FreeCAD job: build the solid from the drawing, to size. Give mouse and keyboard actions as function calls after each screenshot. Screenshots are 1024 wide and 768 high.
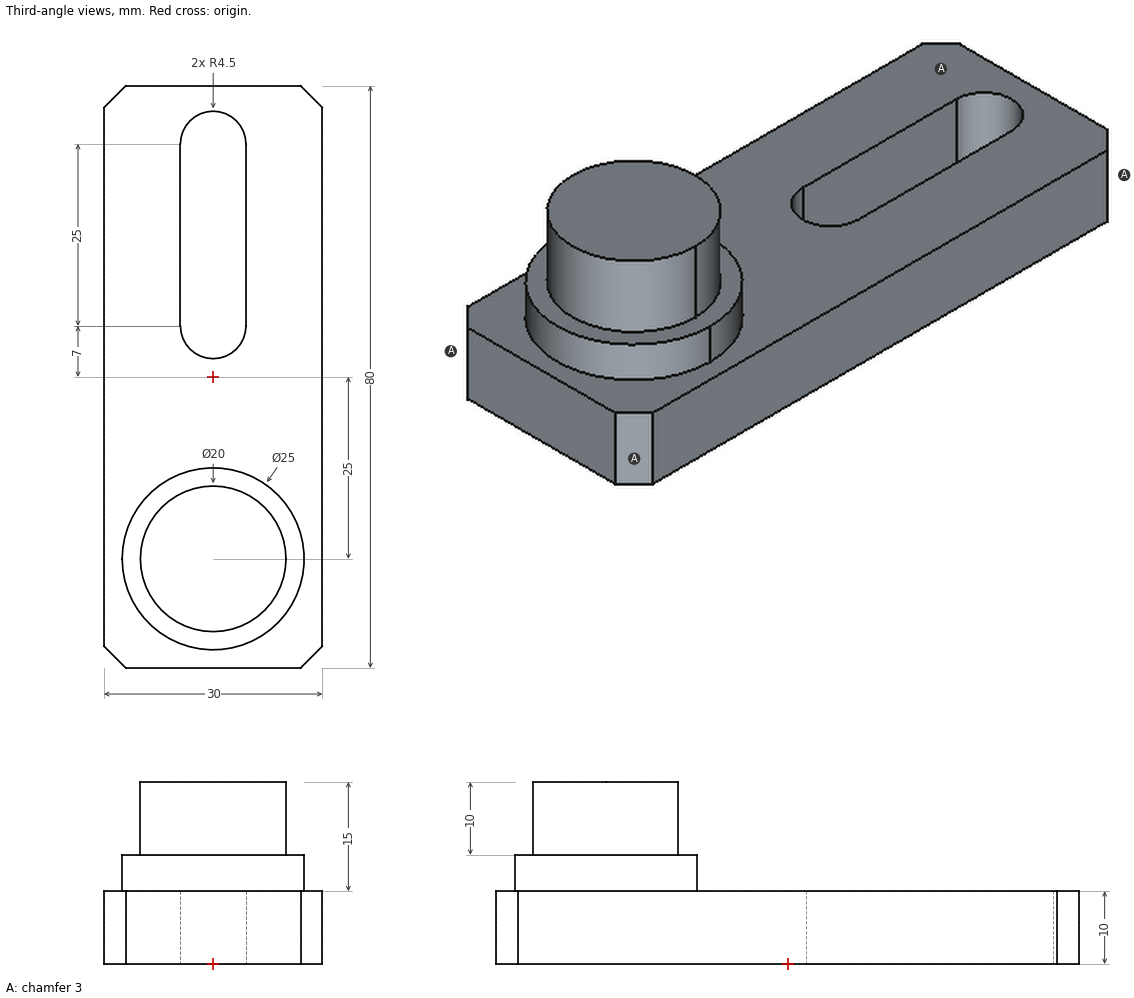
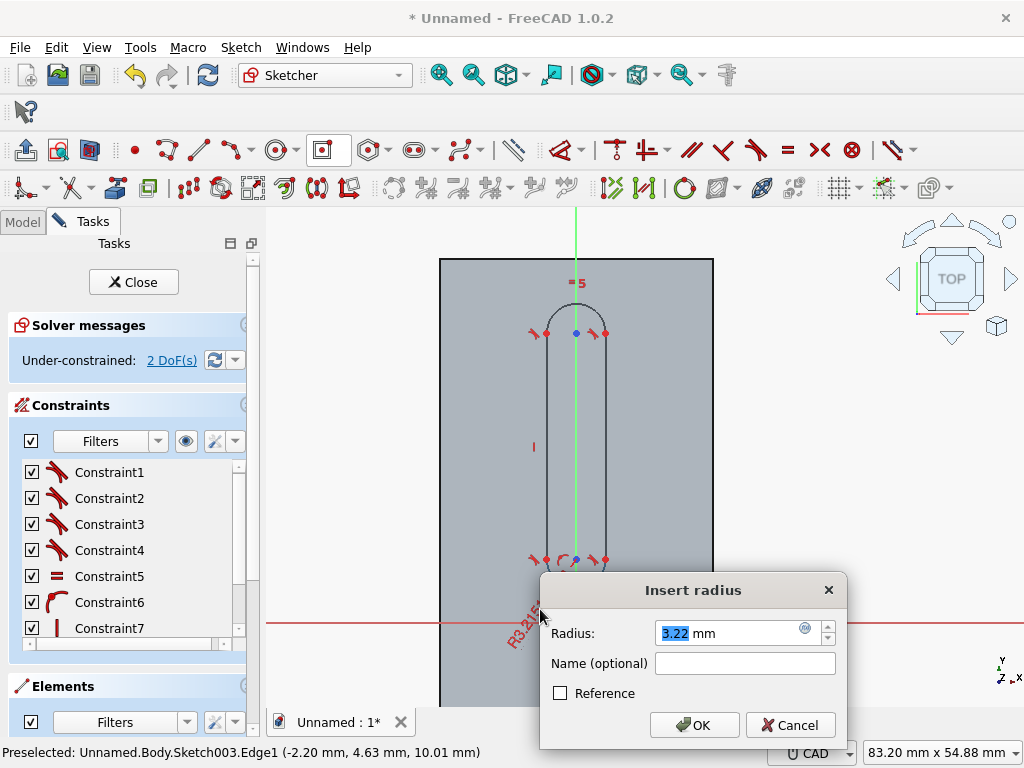
text(4.5)
key(Return)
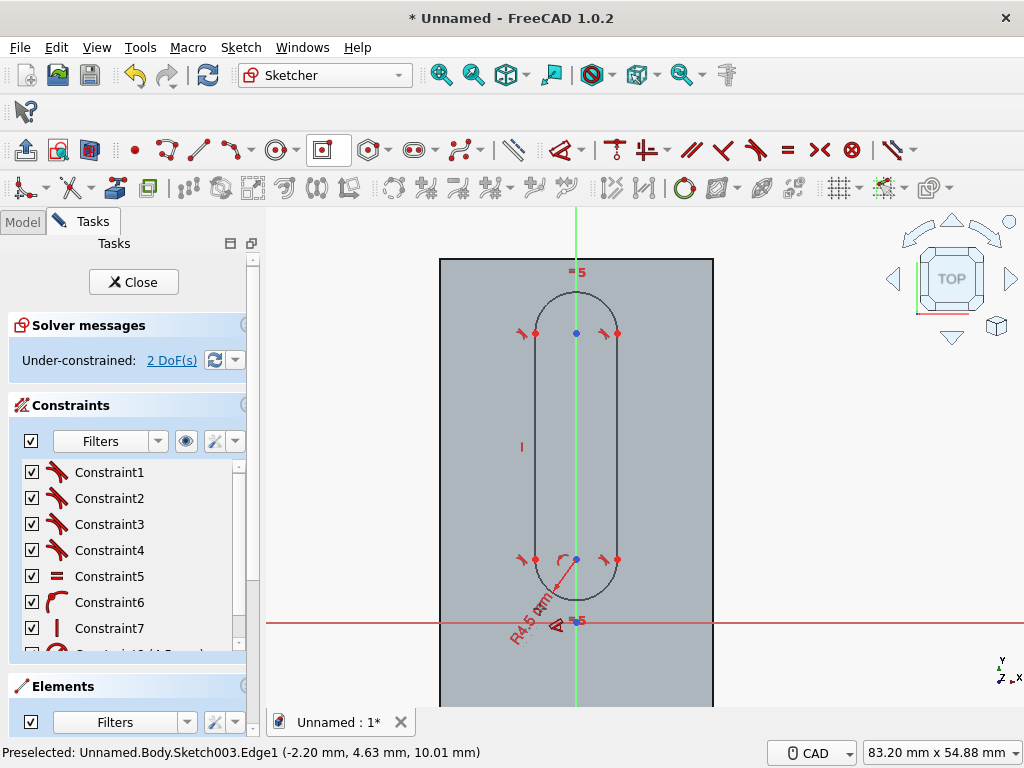
click(535, 492)
click(501, 446)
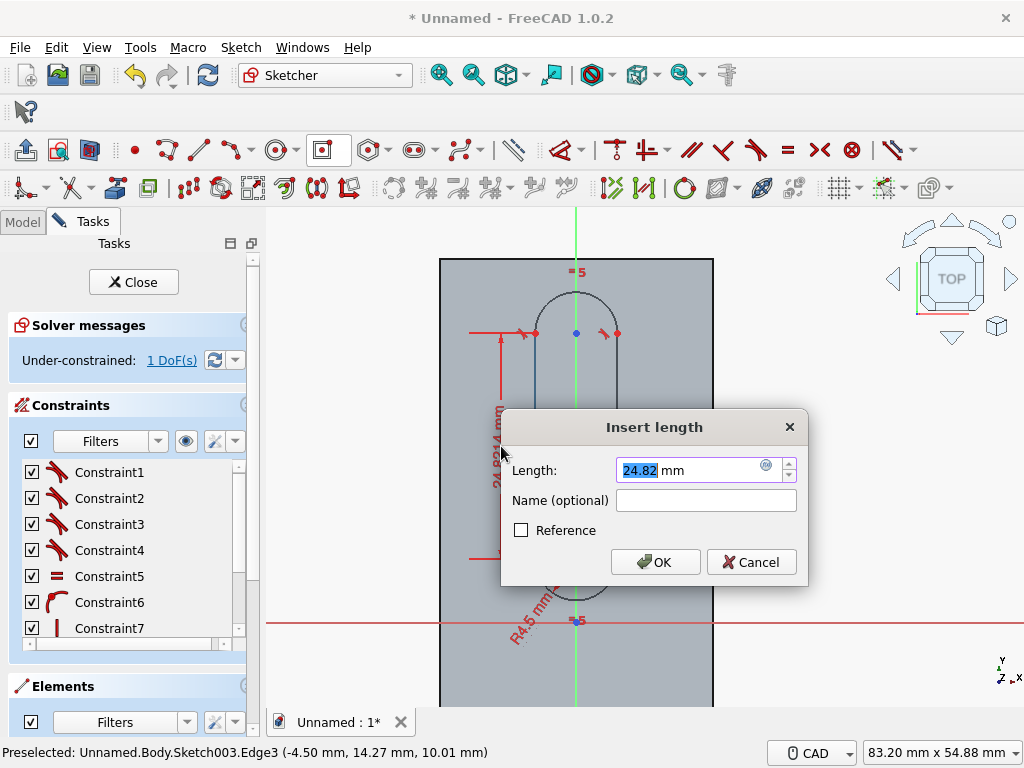
text(25)
key(Return)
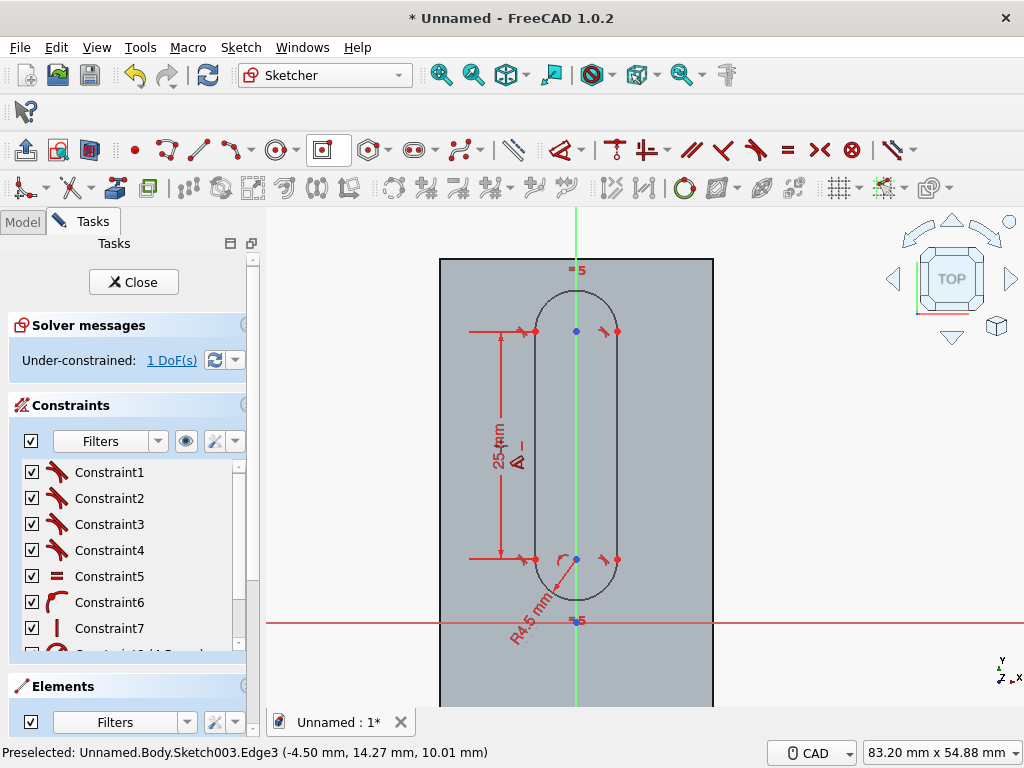
click(535, 559)
click(501, 577)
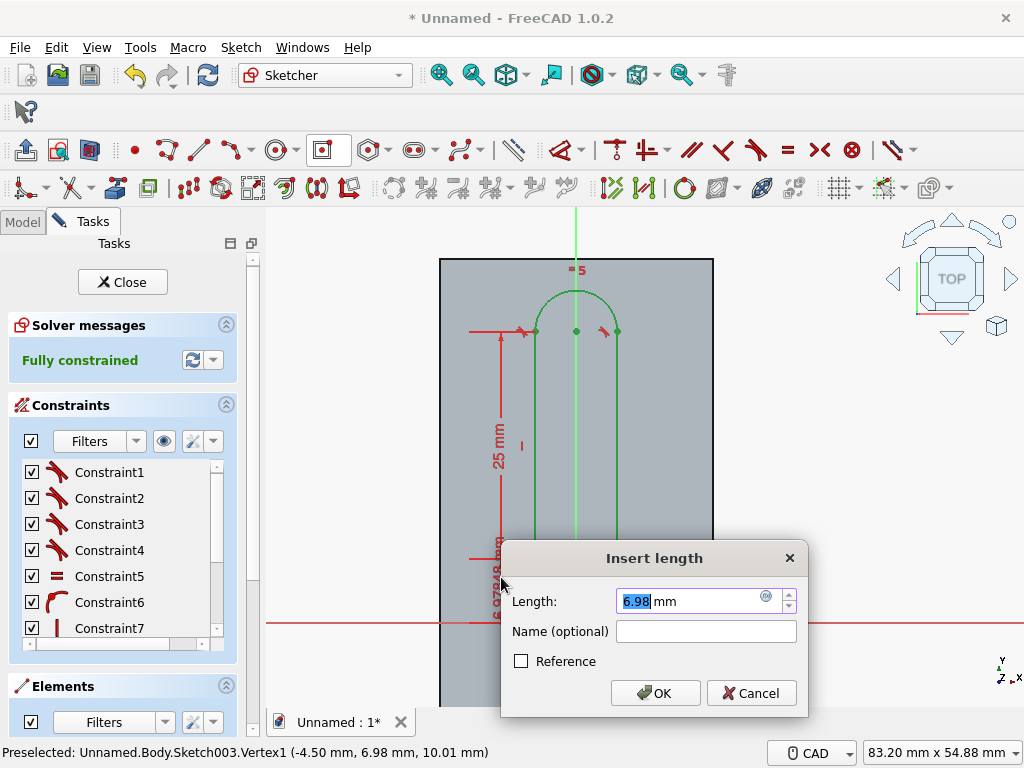
text(7)
key(Return)
key(Escape)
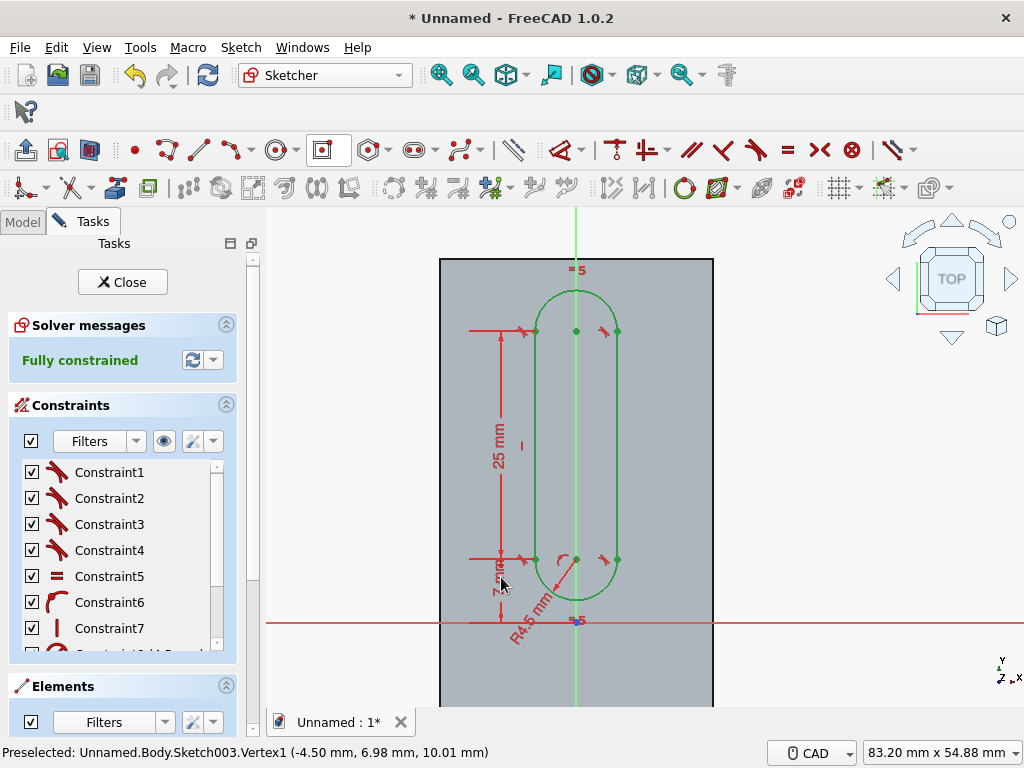
click(123, 282)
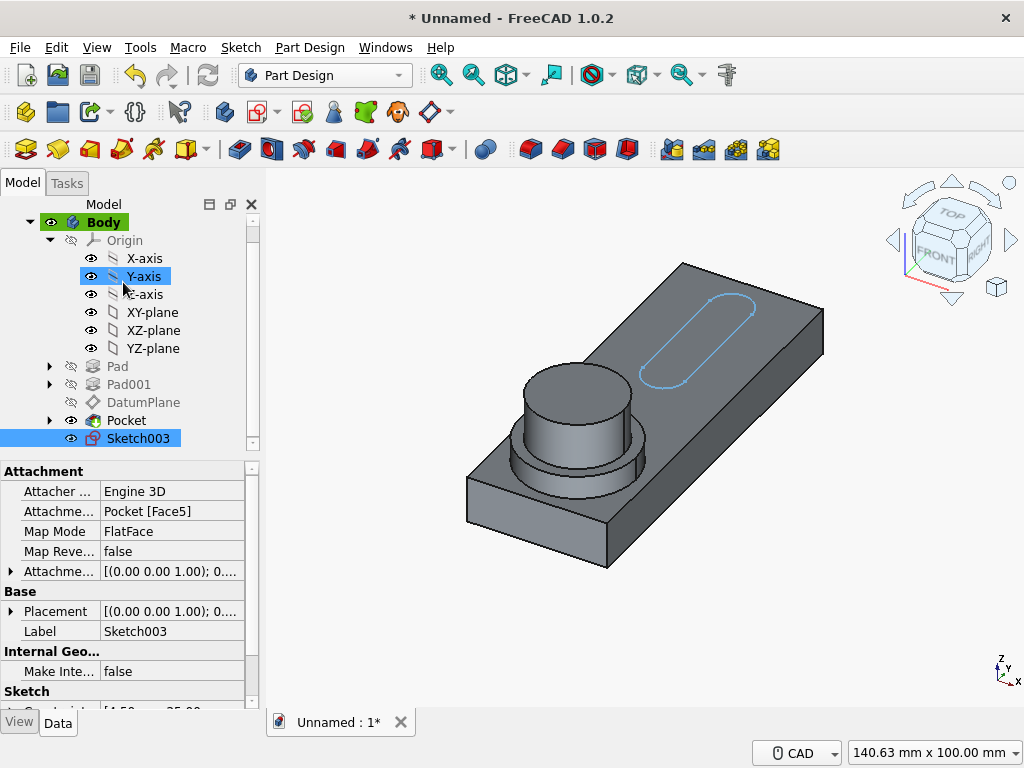
click(240, 150)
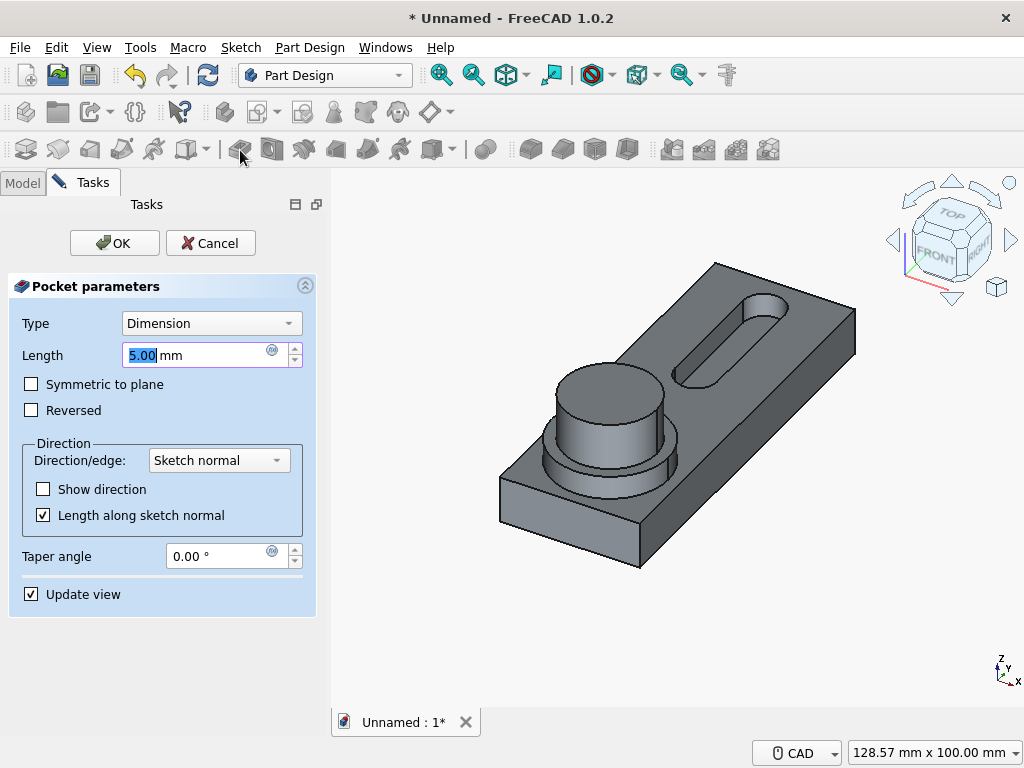
click(212, 324)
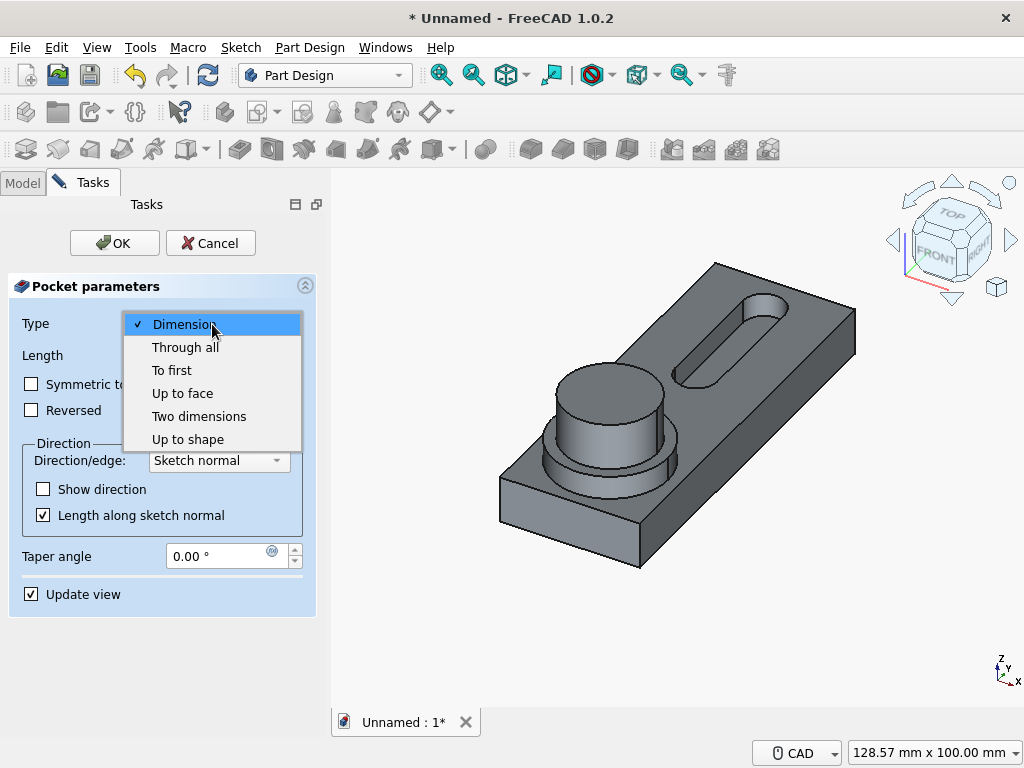
click(212, 348)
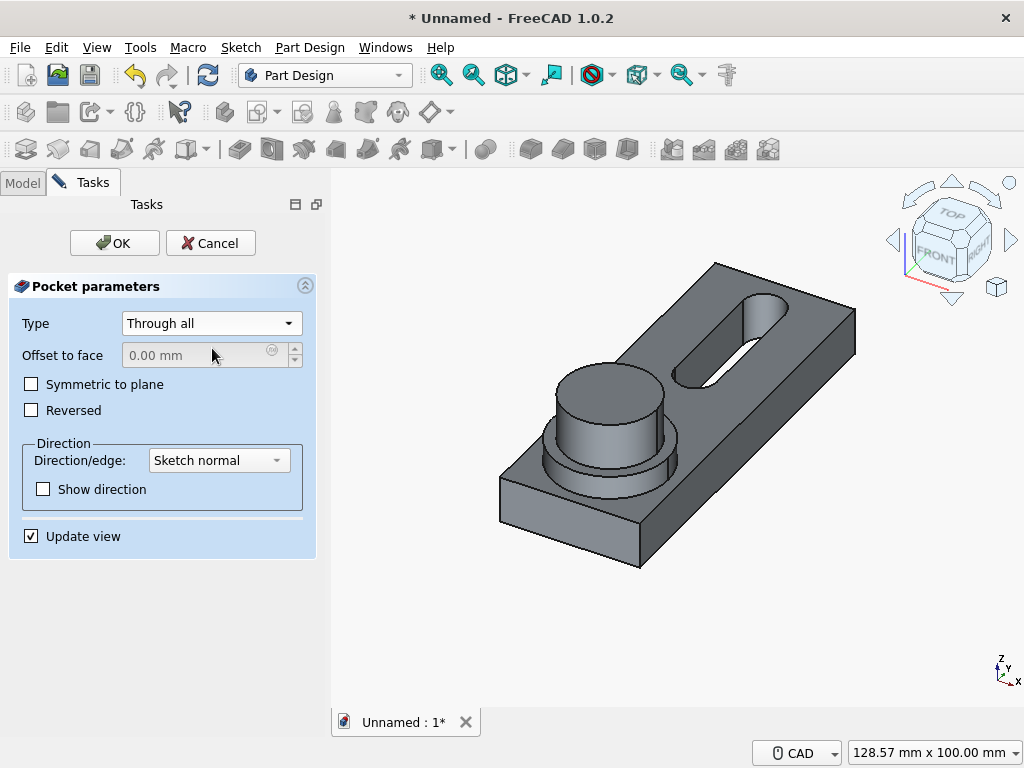
click(115, 243)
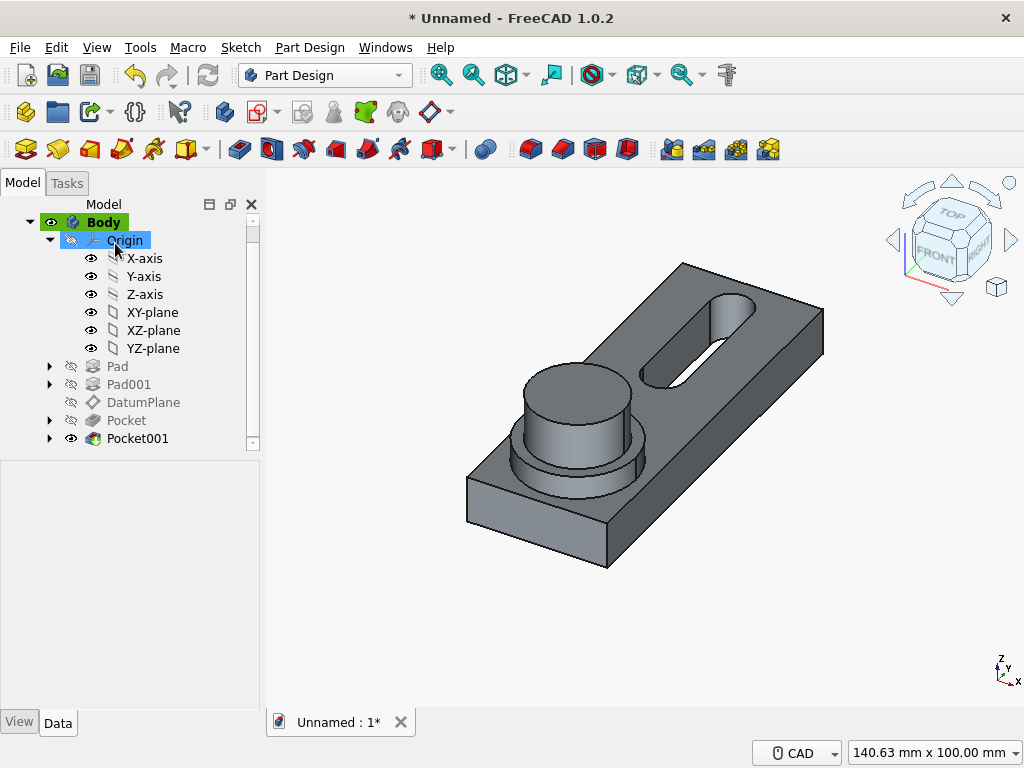
click(607, 545)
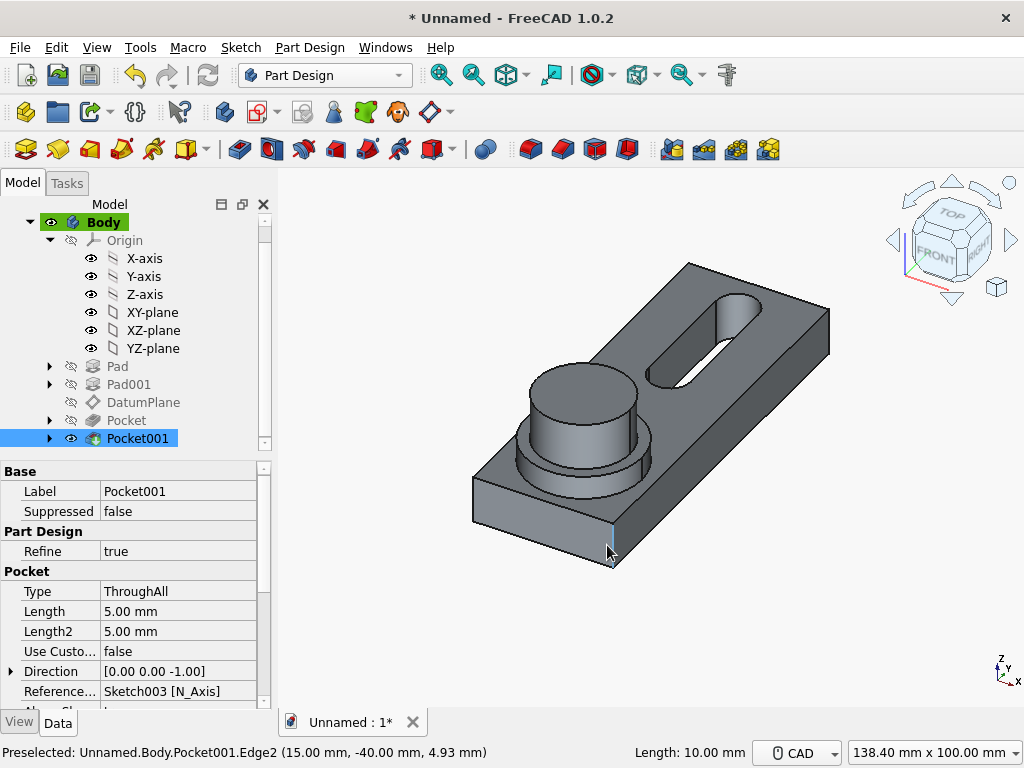
key(0)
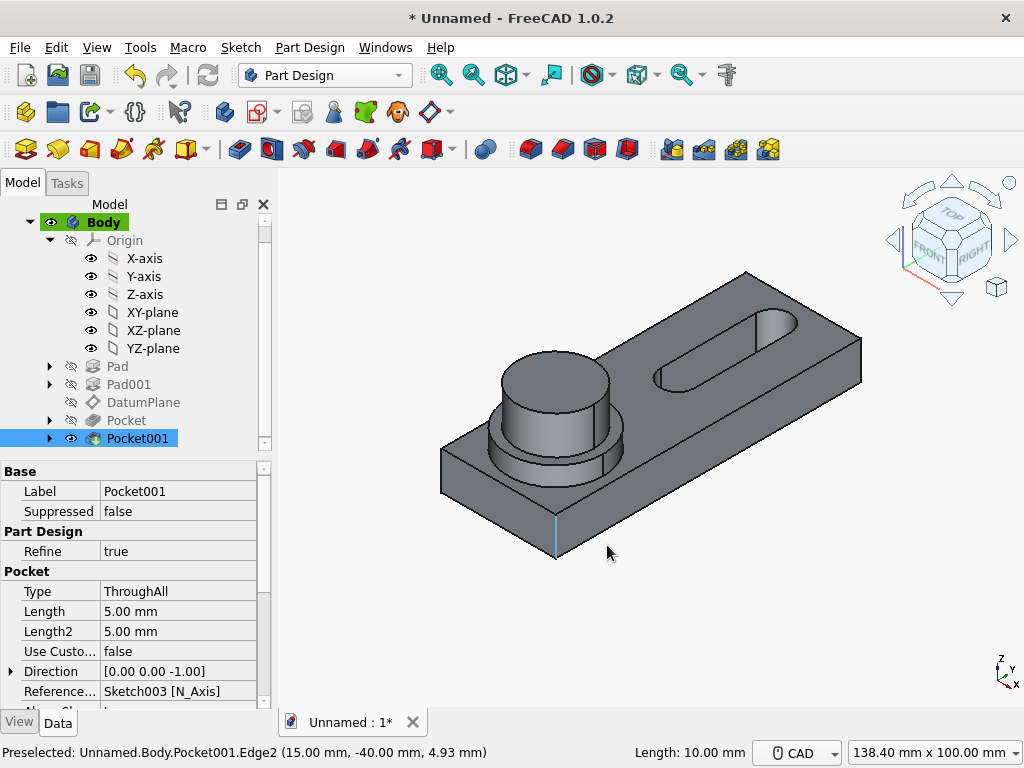
key(2)